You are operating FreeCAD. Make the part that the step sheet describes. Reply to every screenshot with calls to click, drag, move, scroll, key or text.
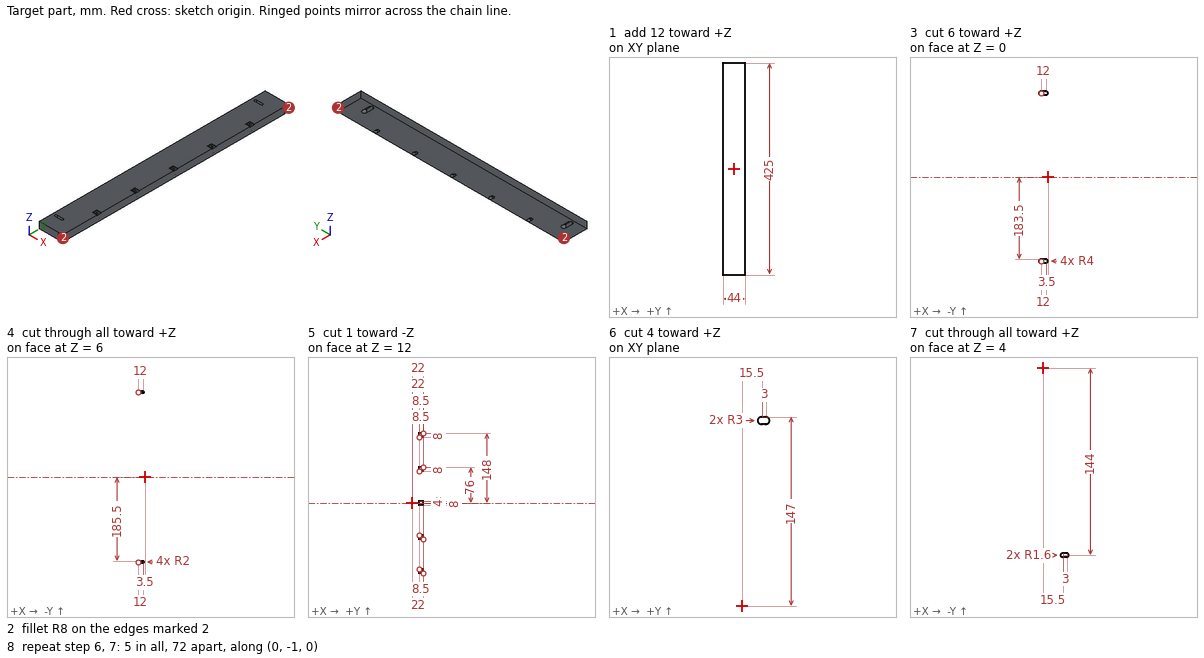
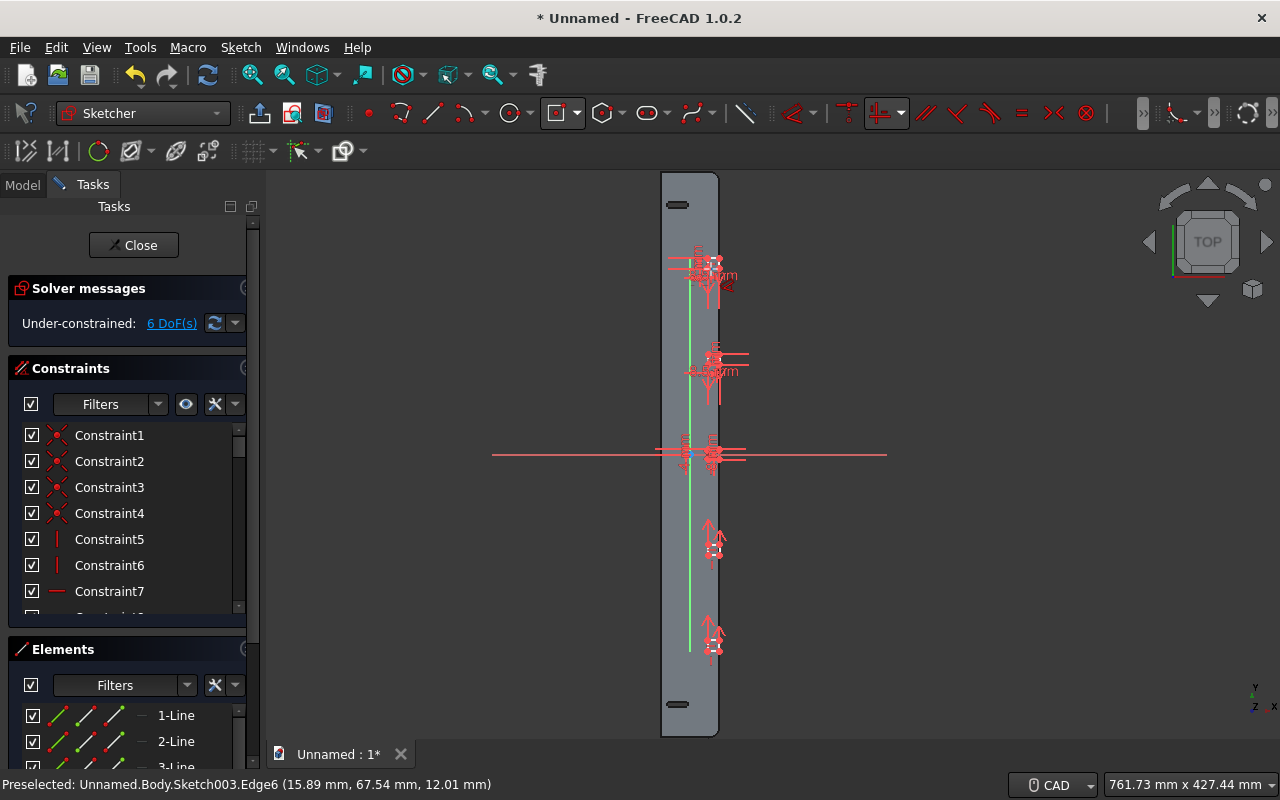
scroll(712, 460, up, 8)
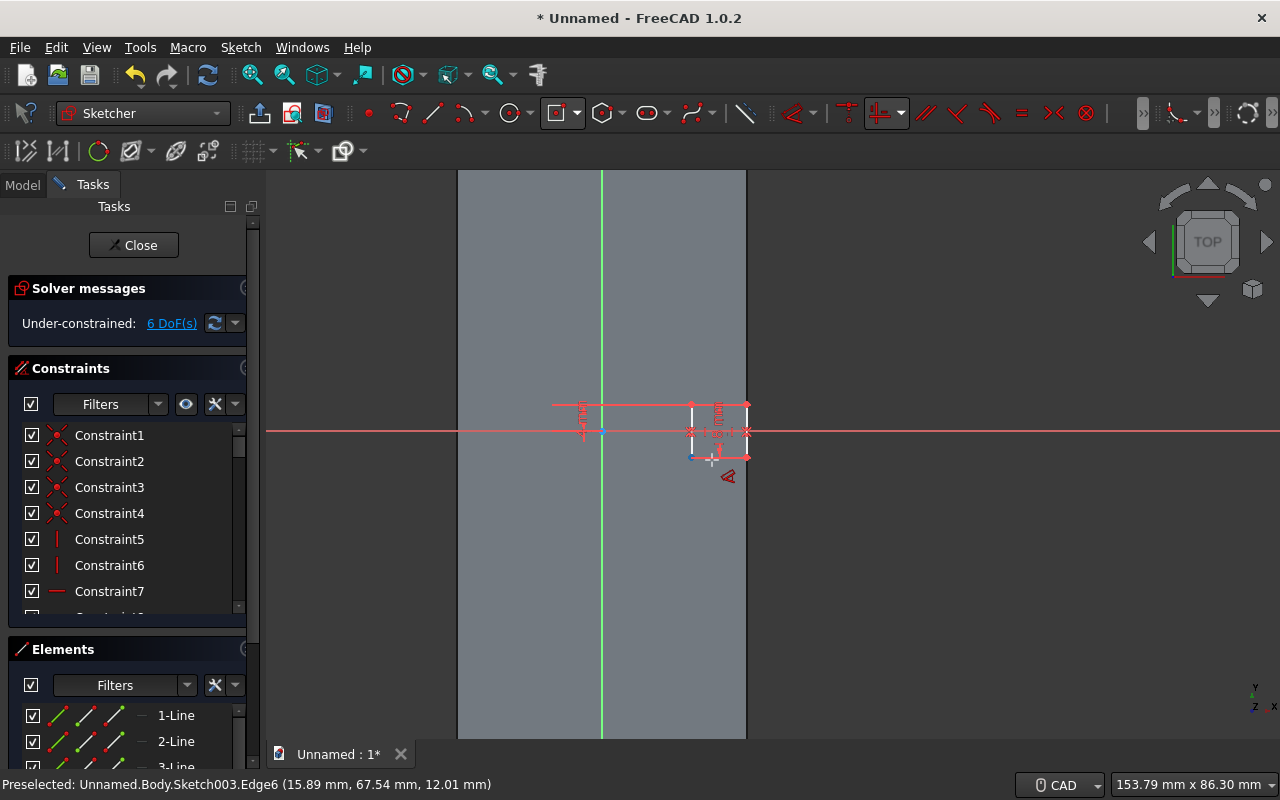
click(708, 458)
click(719, 492)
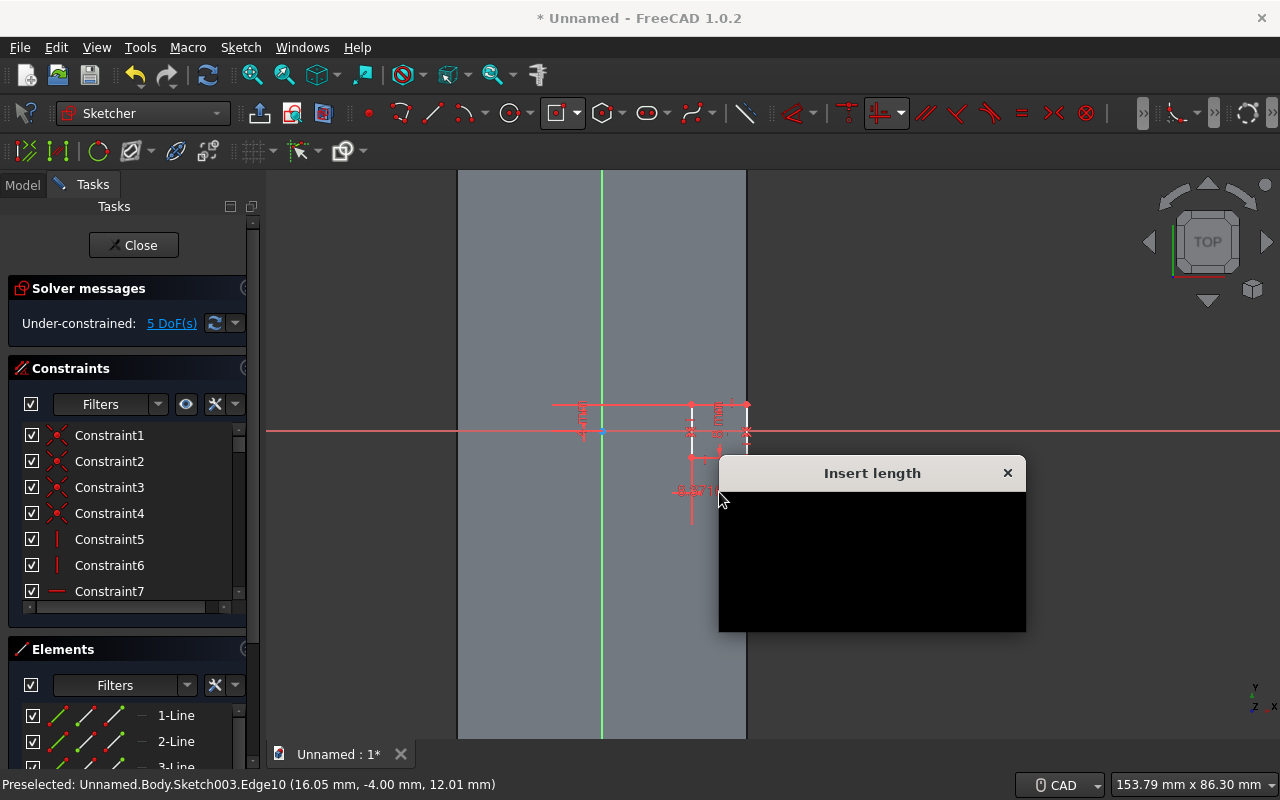
text(8.5)
key(Return)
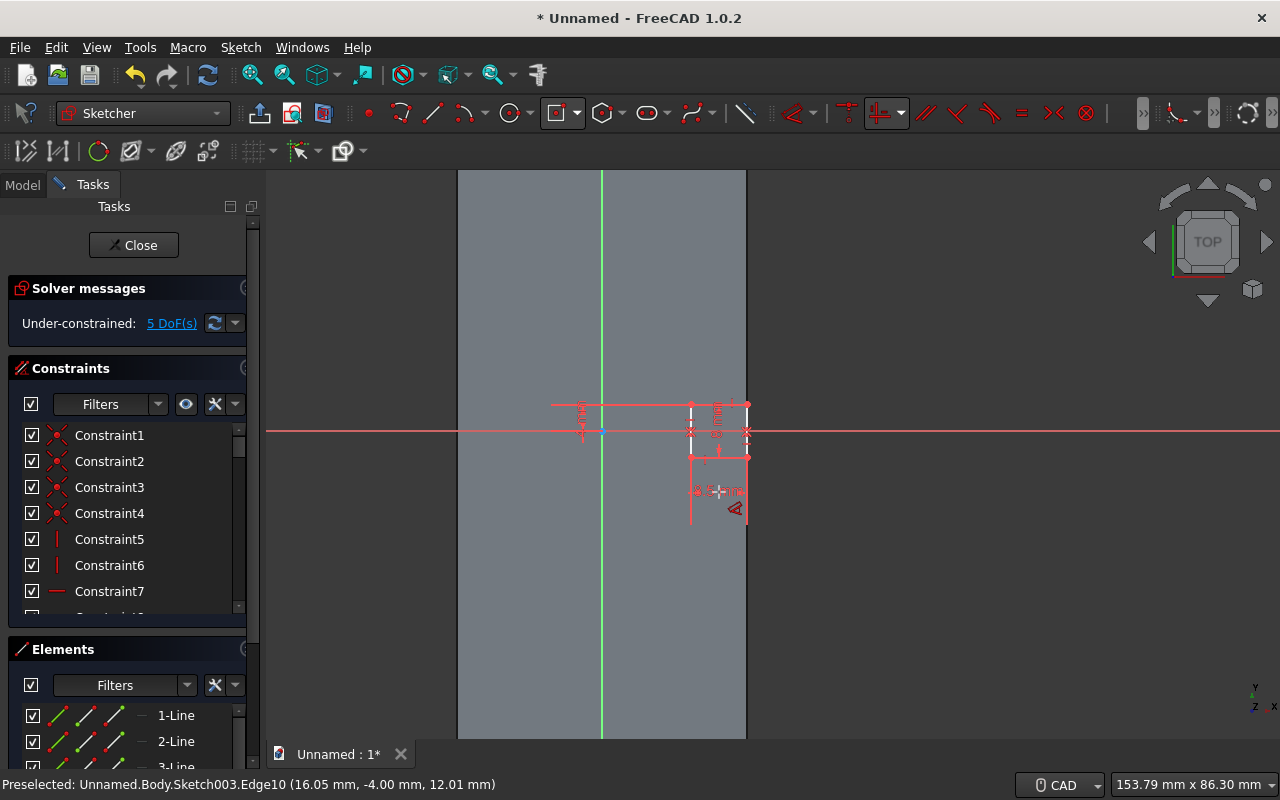
scroll(712, 460, down, 8)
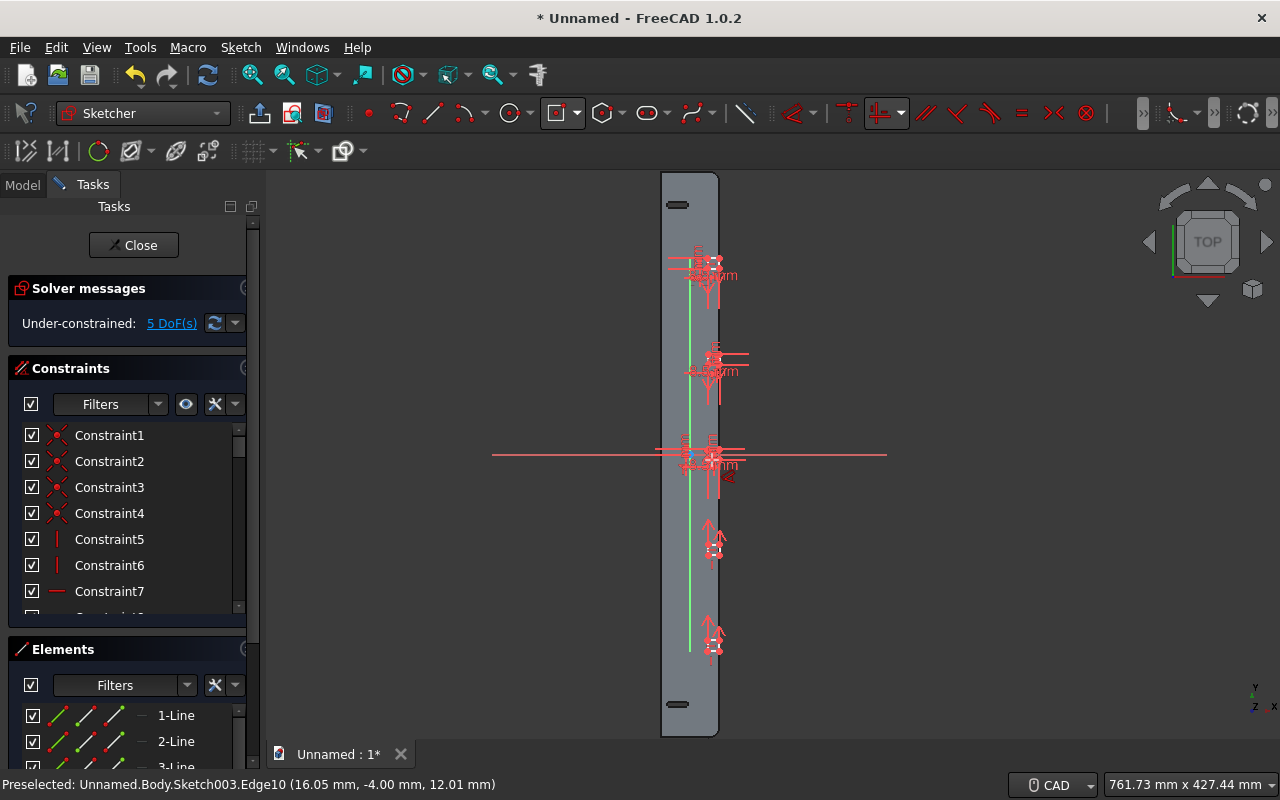
scroll(719, 269, up, 2)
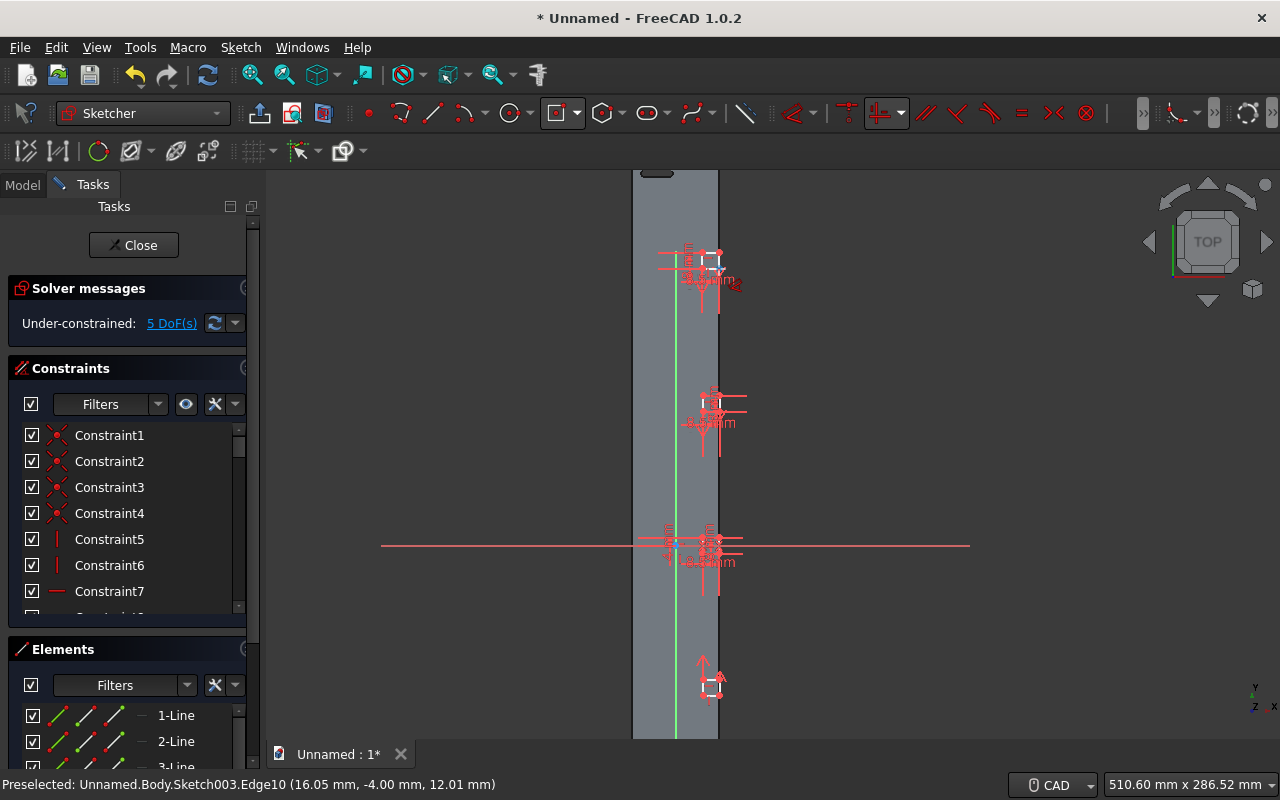
click(719, 269)
click(697, 235)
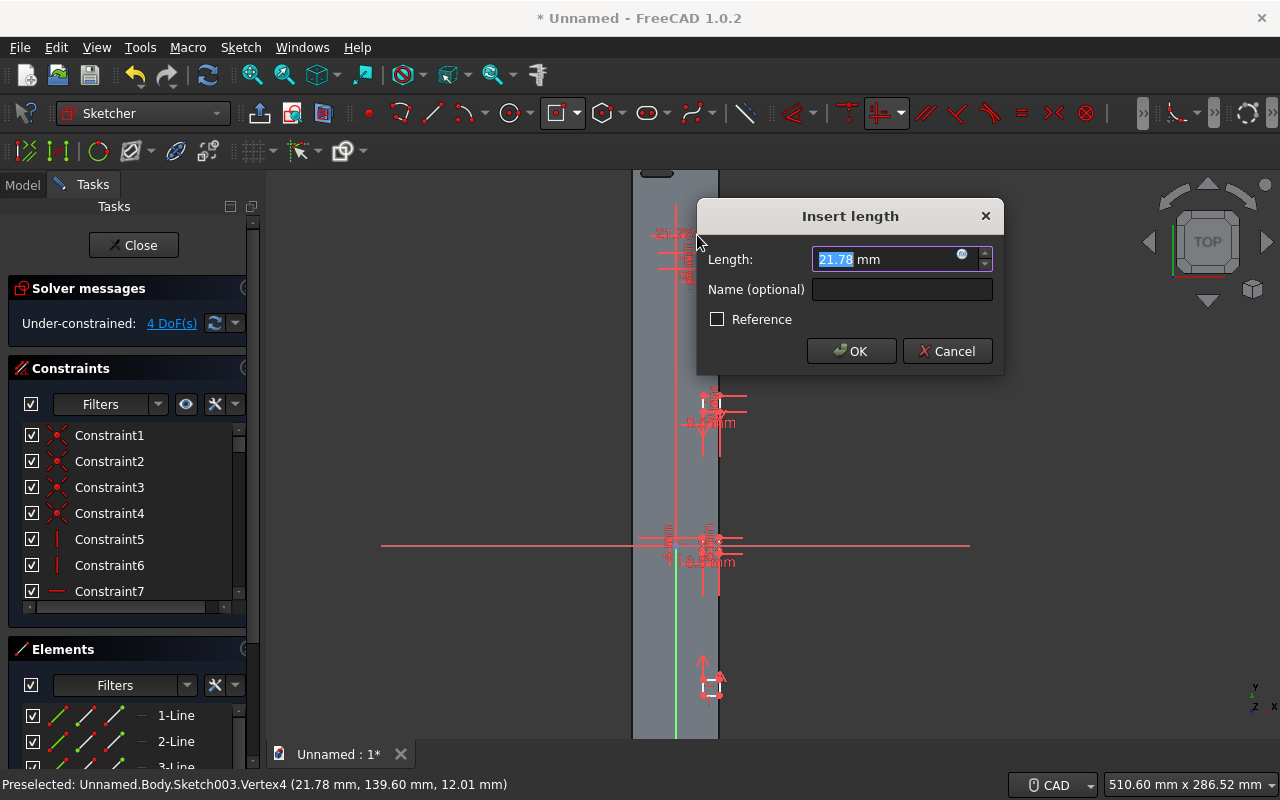
text(22)
key(Return)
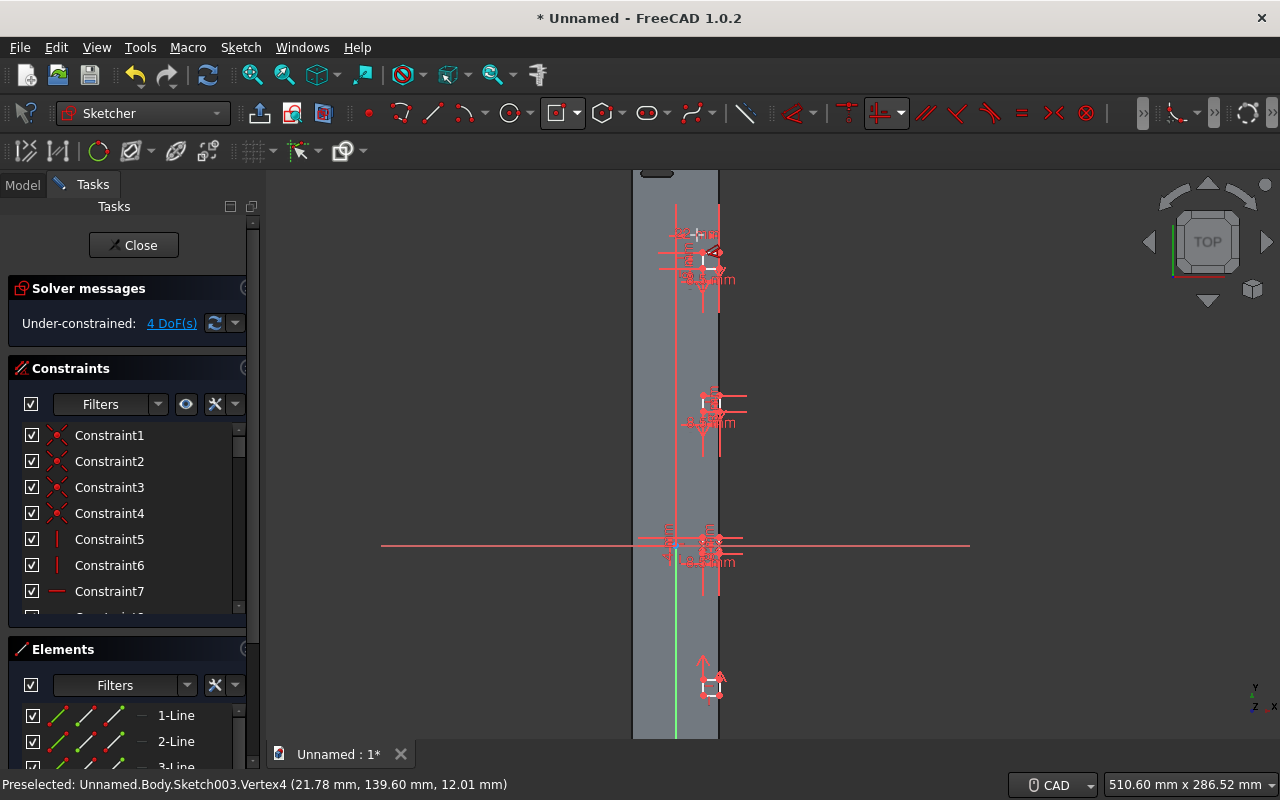
click(703, 396)
click(642, 471)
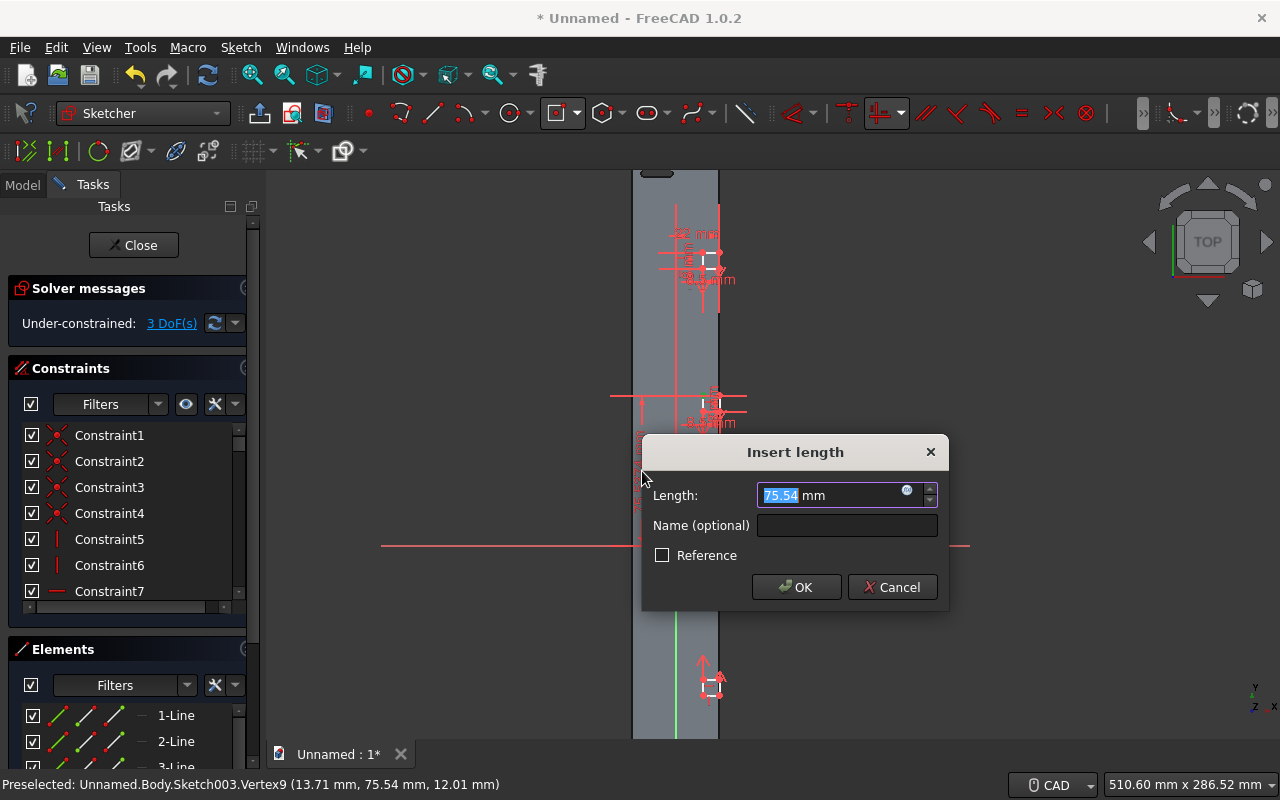
text(76)
key(Return)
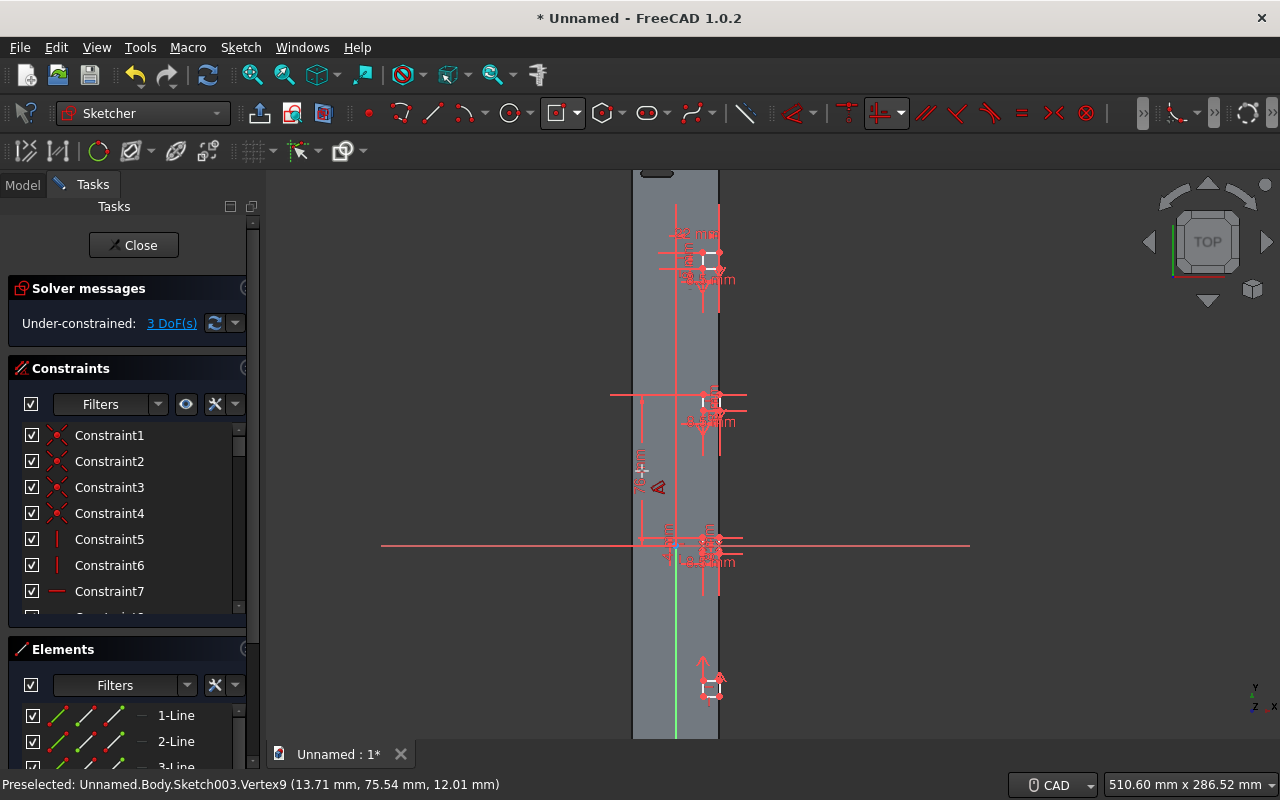
click(720, 411)
click(698, 377)